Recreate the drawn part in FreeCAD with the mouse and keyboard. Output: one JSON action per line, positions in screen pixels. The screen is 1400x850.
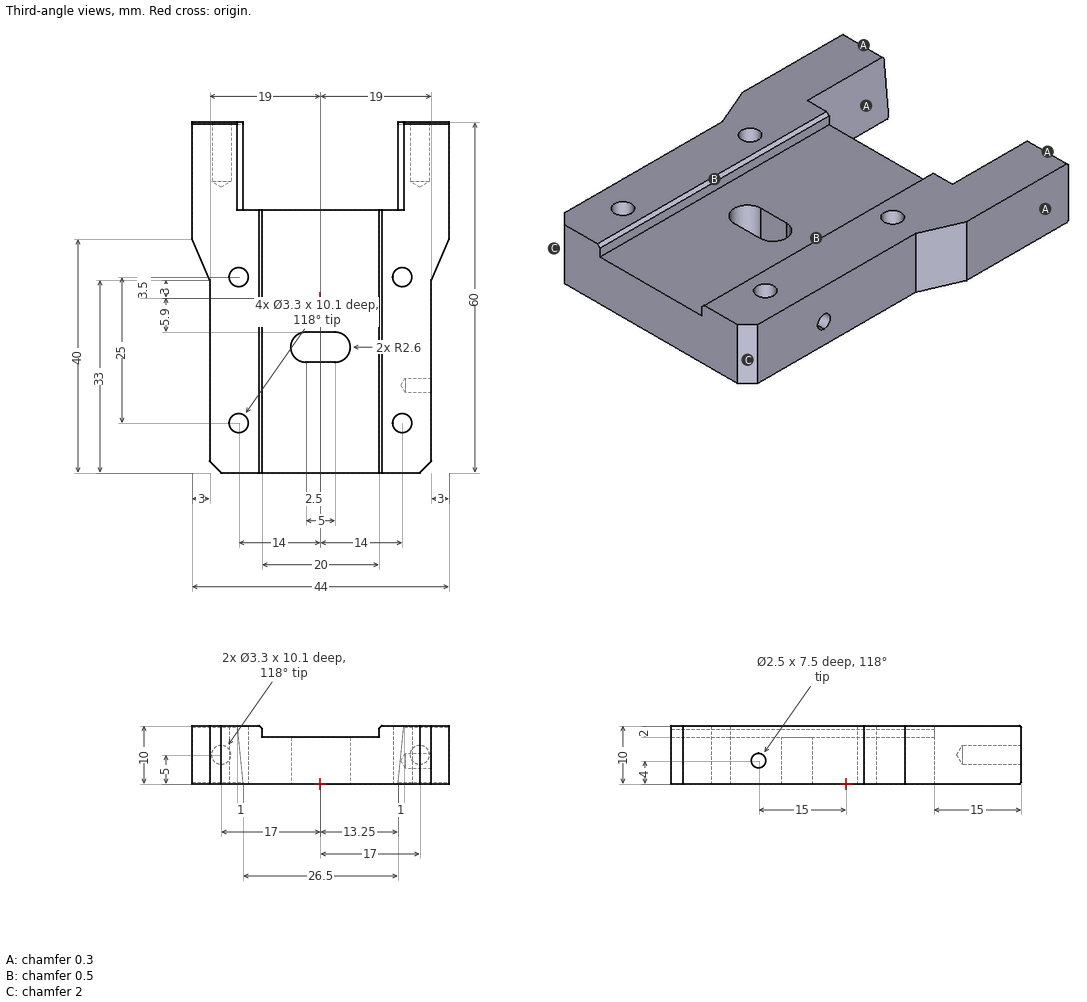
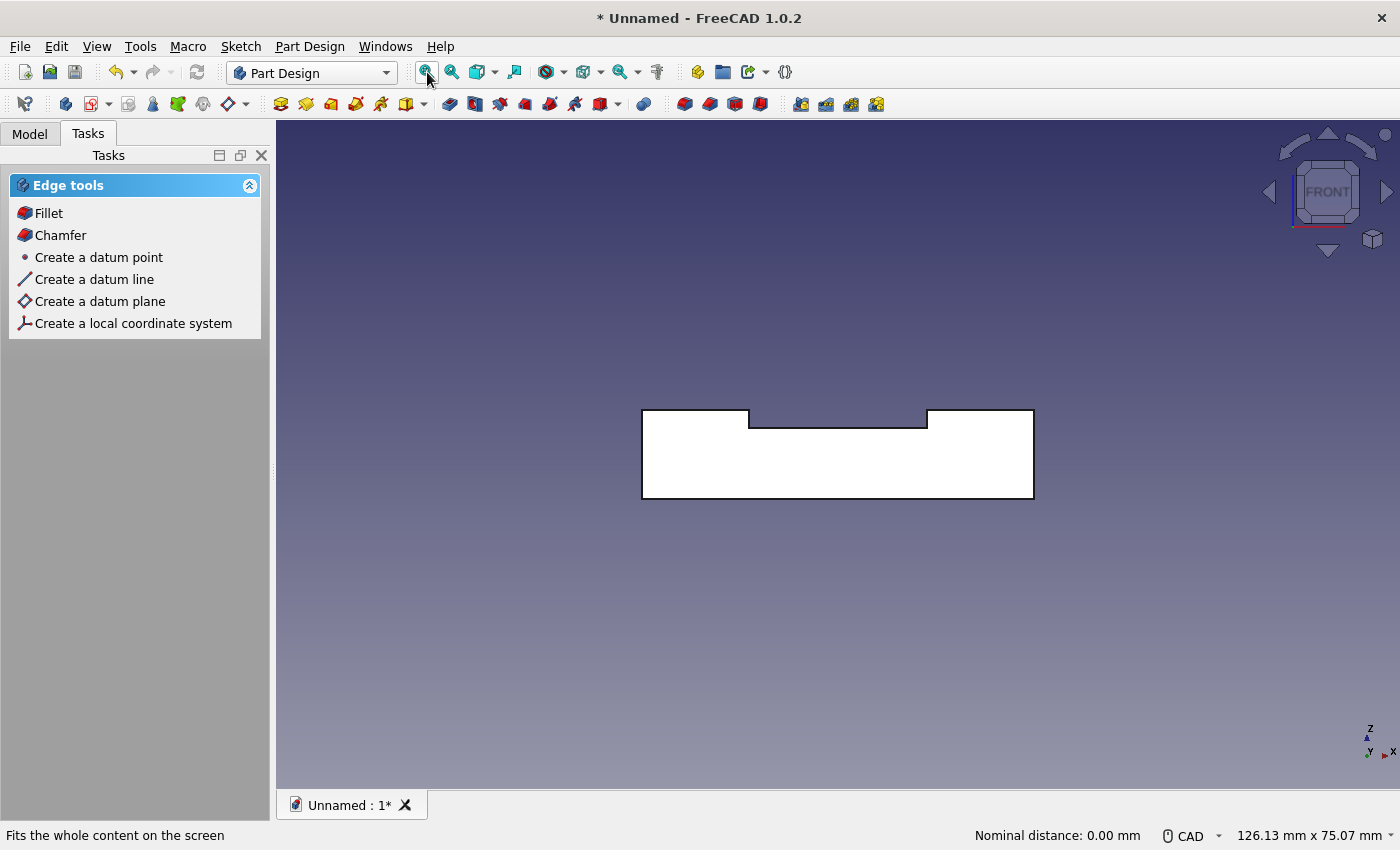
{"action": "key", "text": "3"}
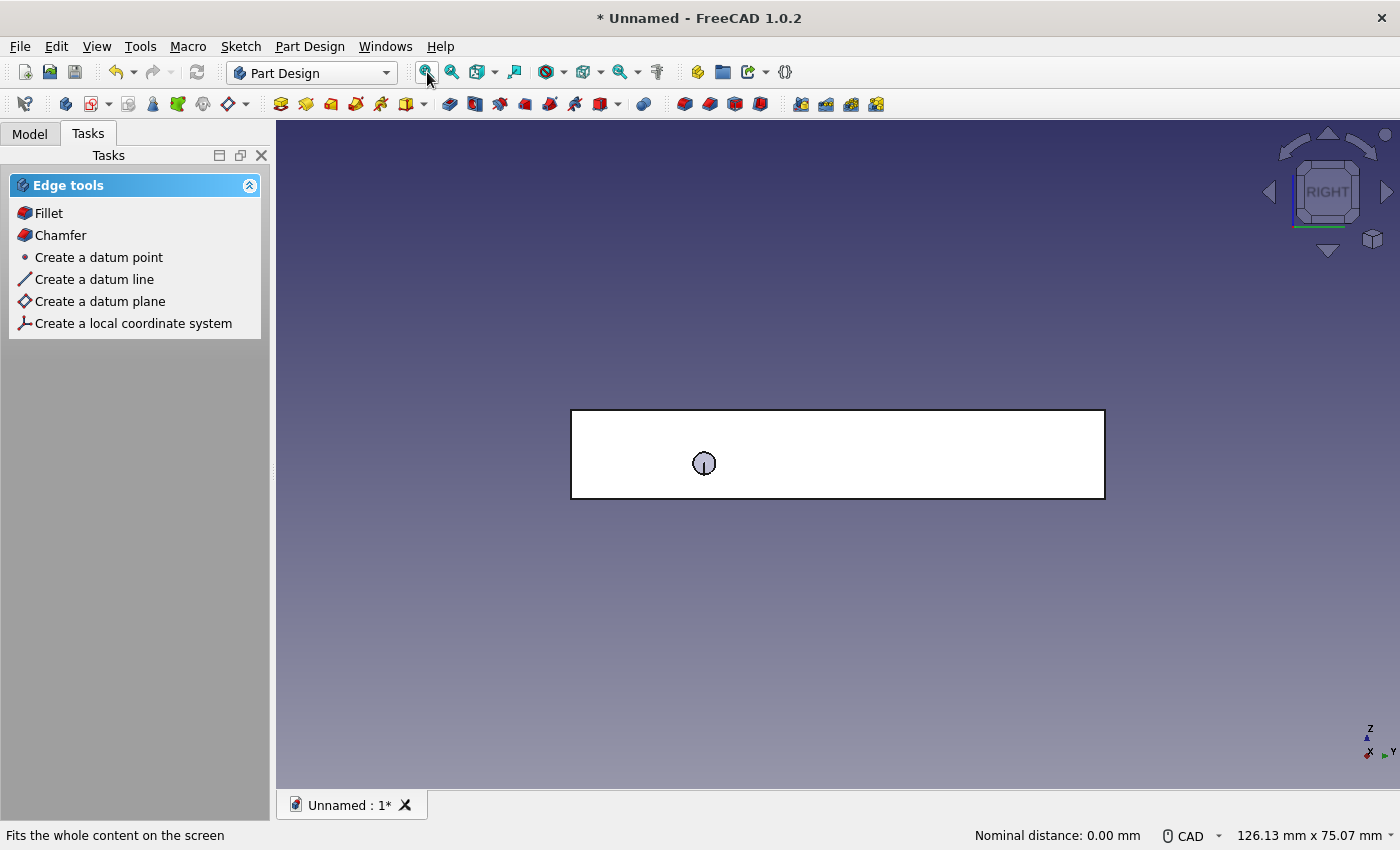
{"action": "key", "text": "5"}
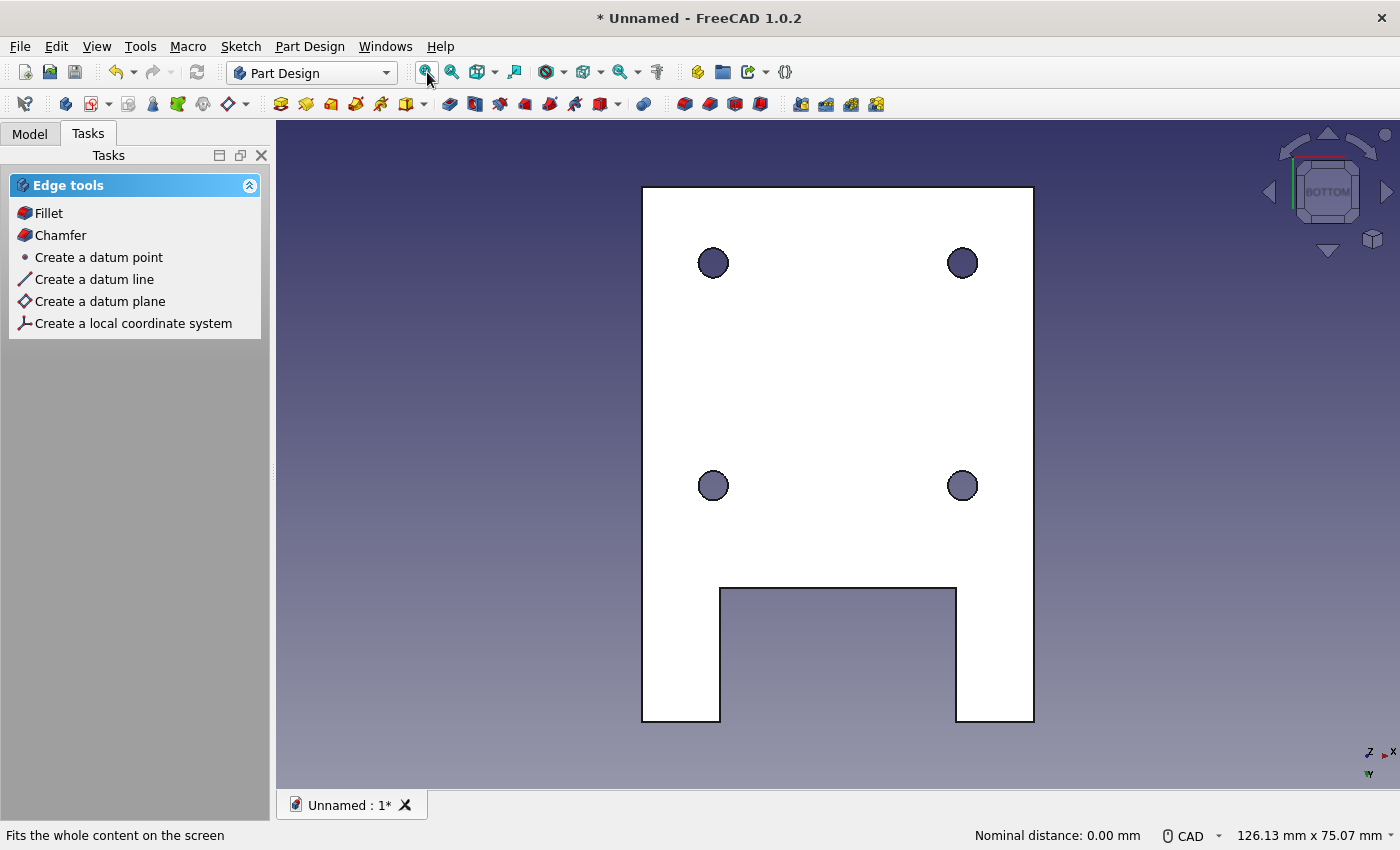
{"action": "left_click", "coordinate": [681, 721], "text": "ctrl"}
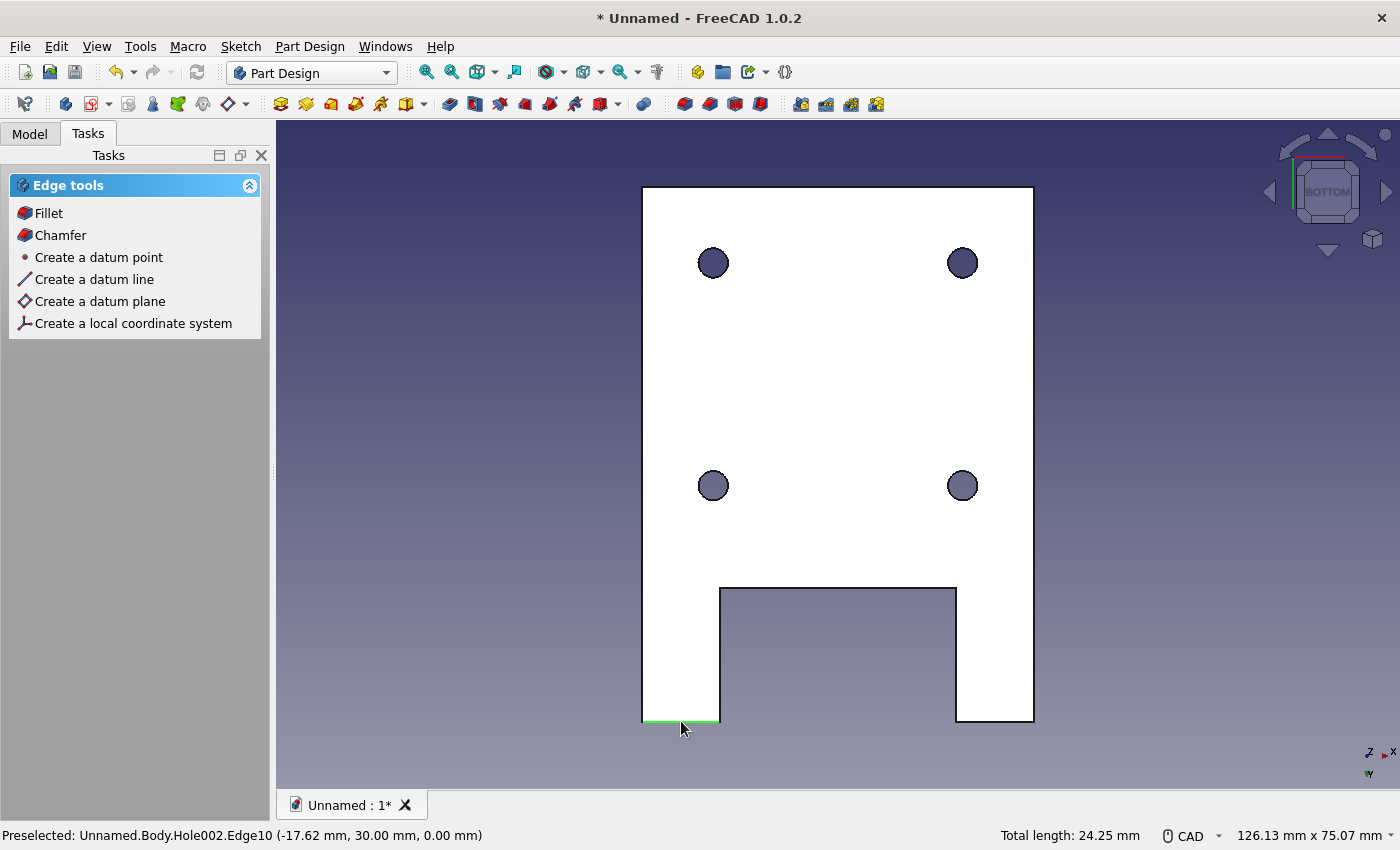
{"action": "left_click", "coordinate": [995, 721], "text": "ctrl"}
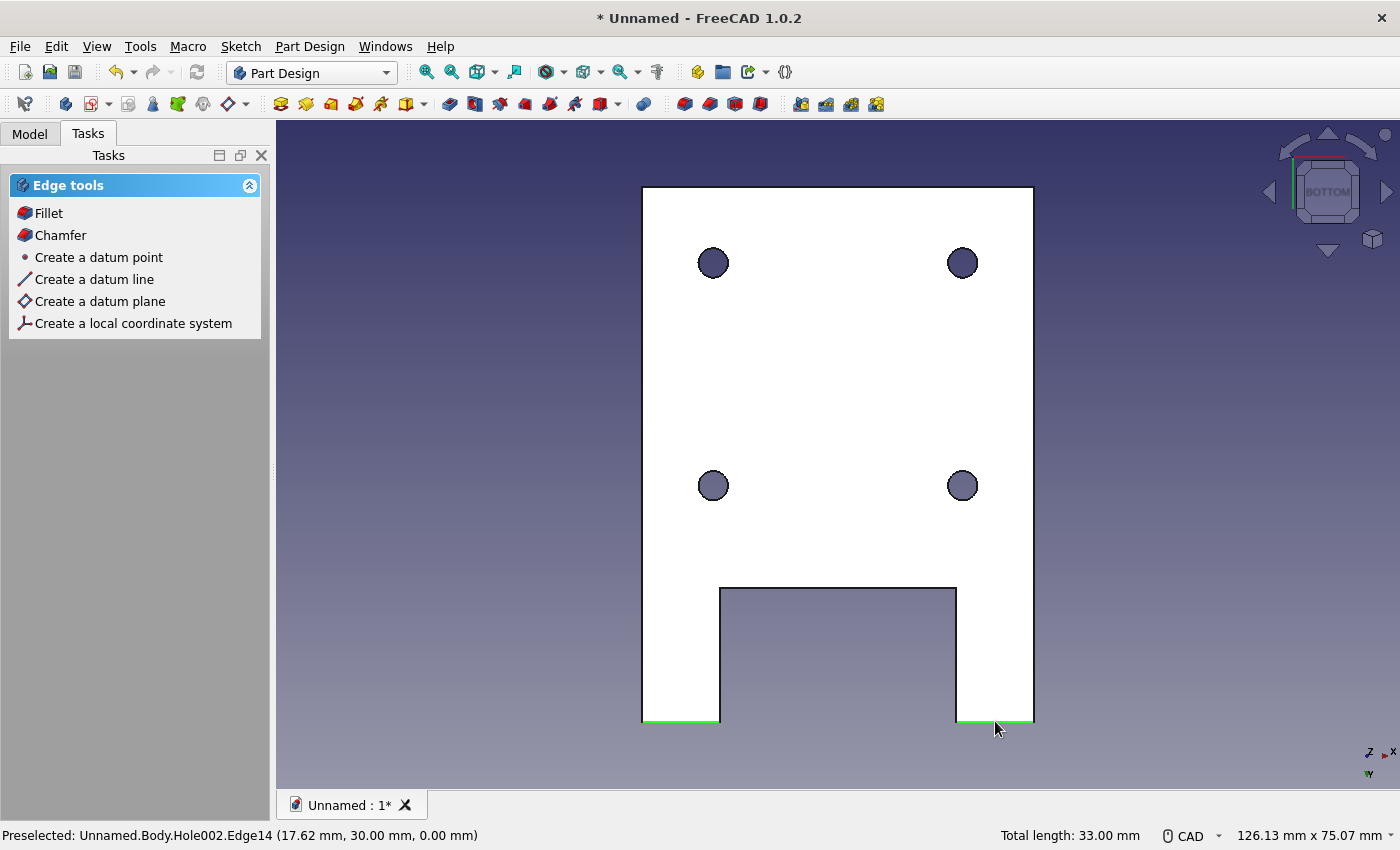
{"action": "left_click", "coordinate": [710, 104]}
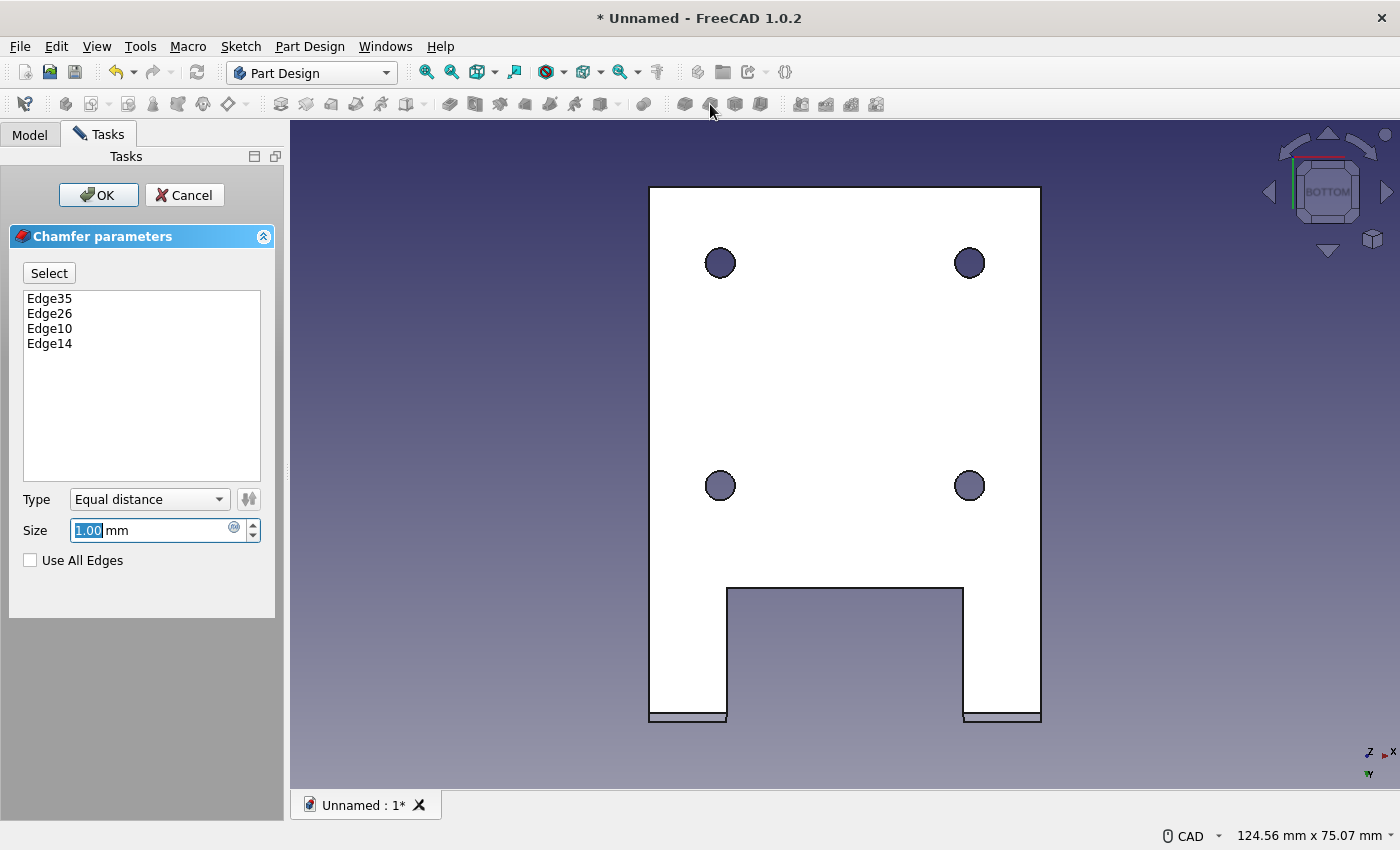
{"action": "type", "text": "0.3"}
{"action": "key", "text": "Tab"}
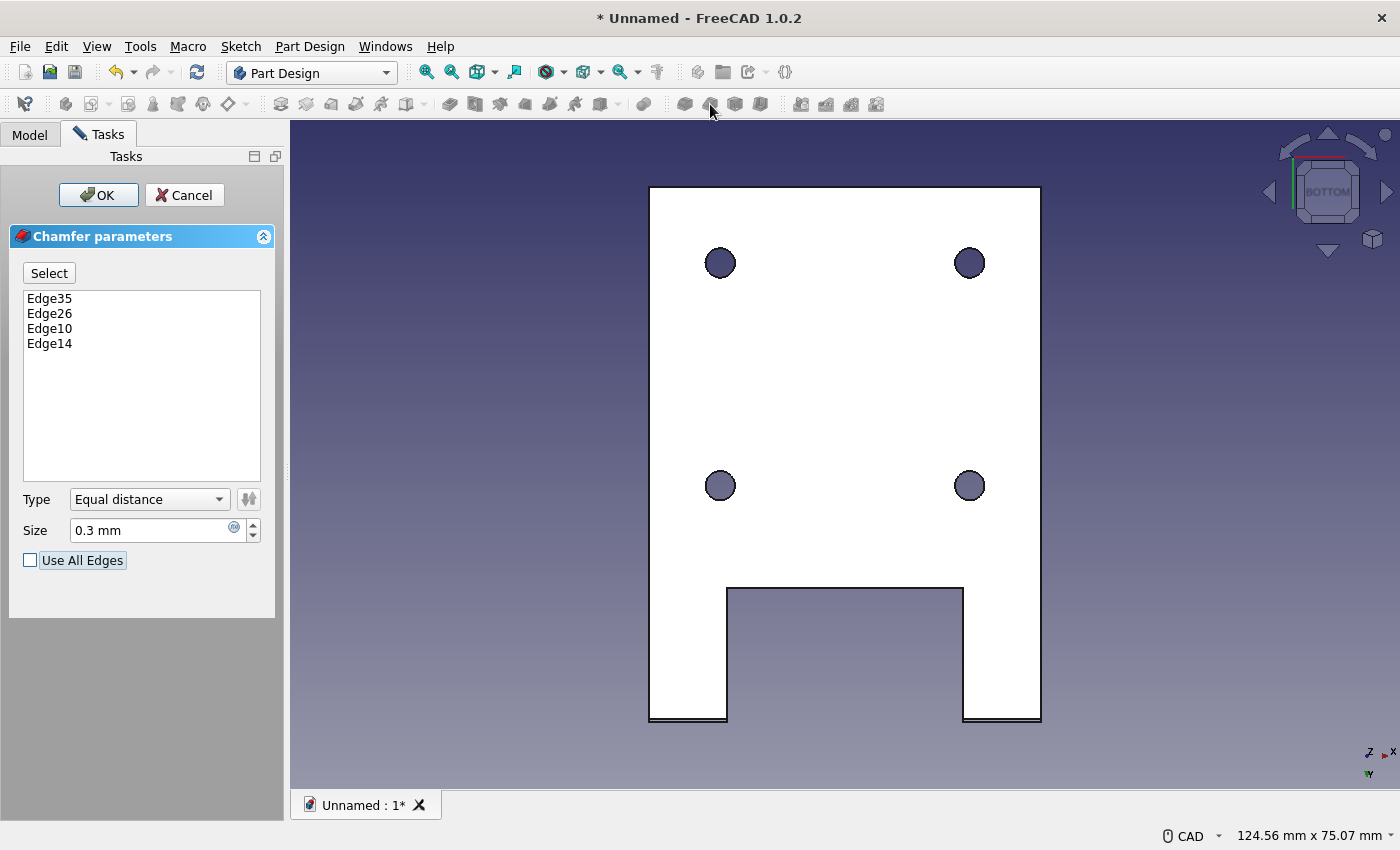
{"action": "left_click", "coordinate": [99, 195]}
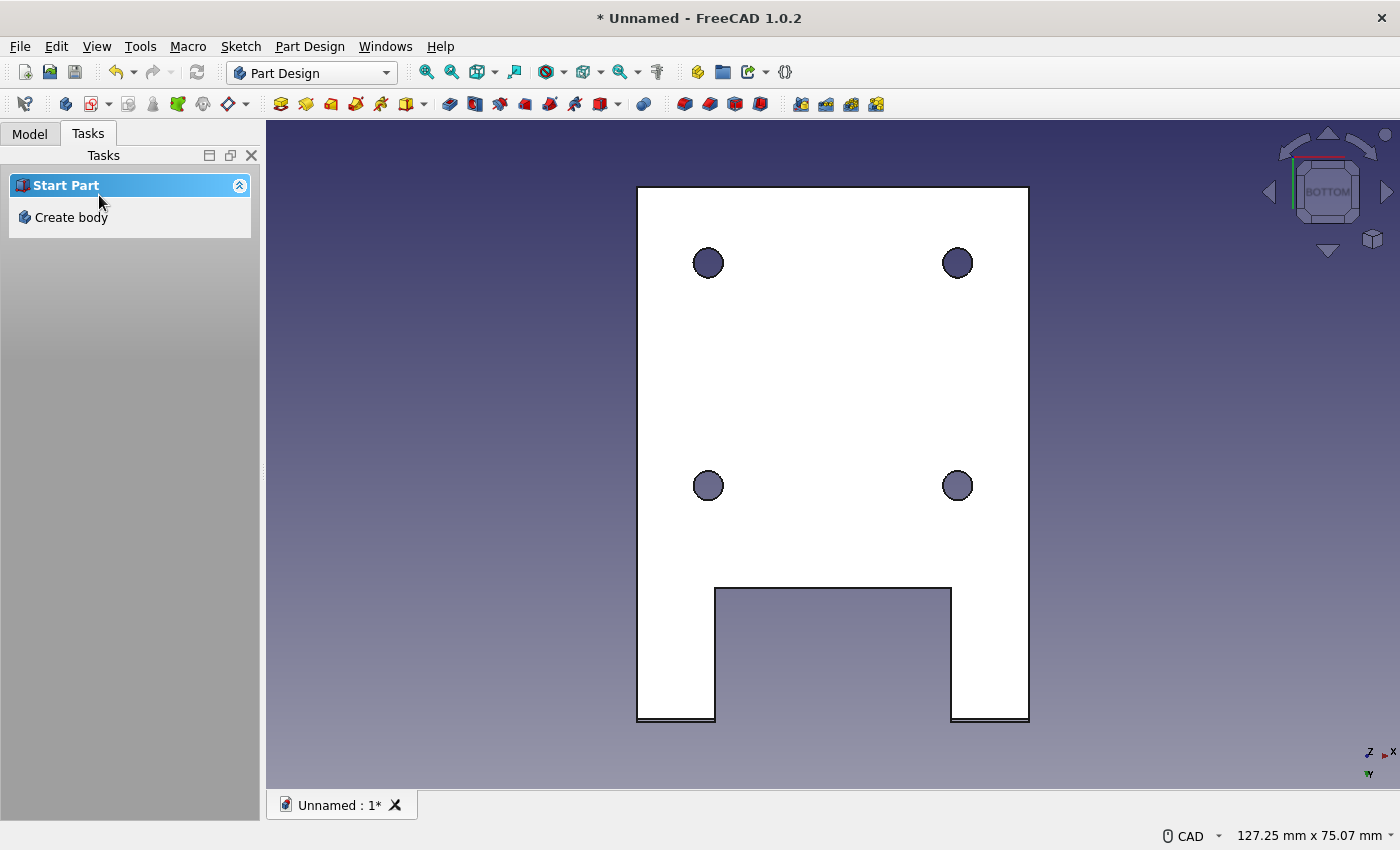
{"action": "key", "text": "0"}